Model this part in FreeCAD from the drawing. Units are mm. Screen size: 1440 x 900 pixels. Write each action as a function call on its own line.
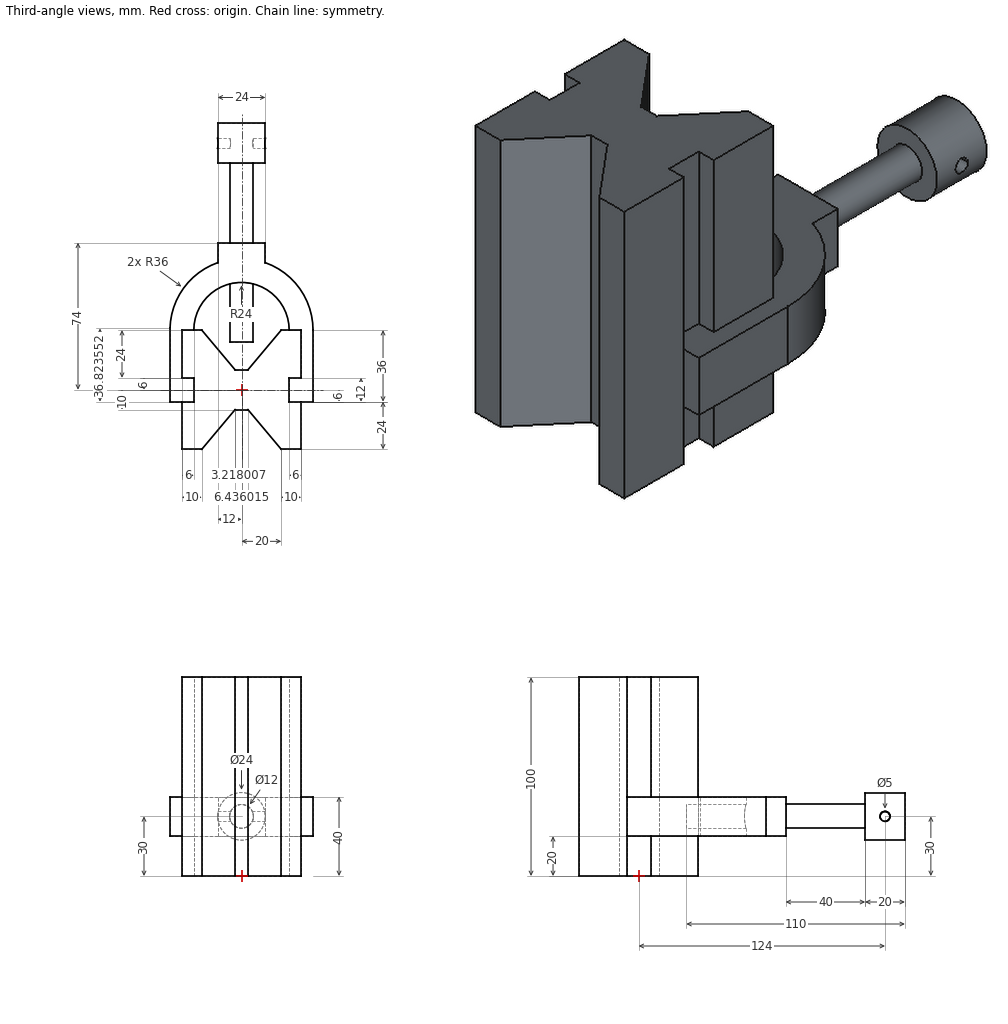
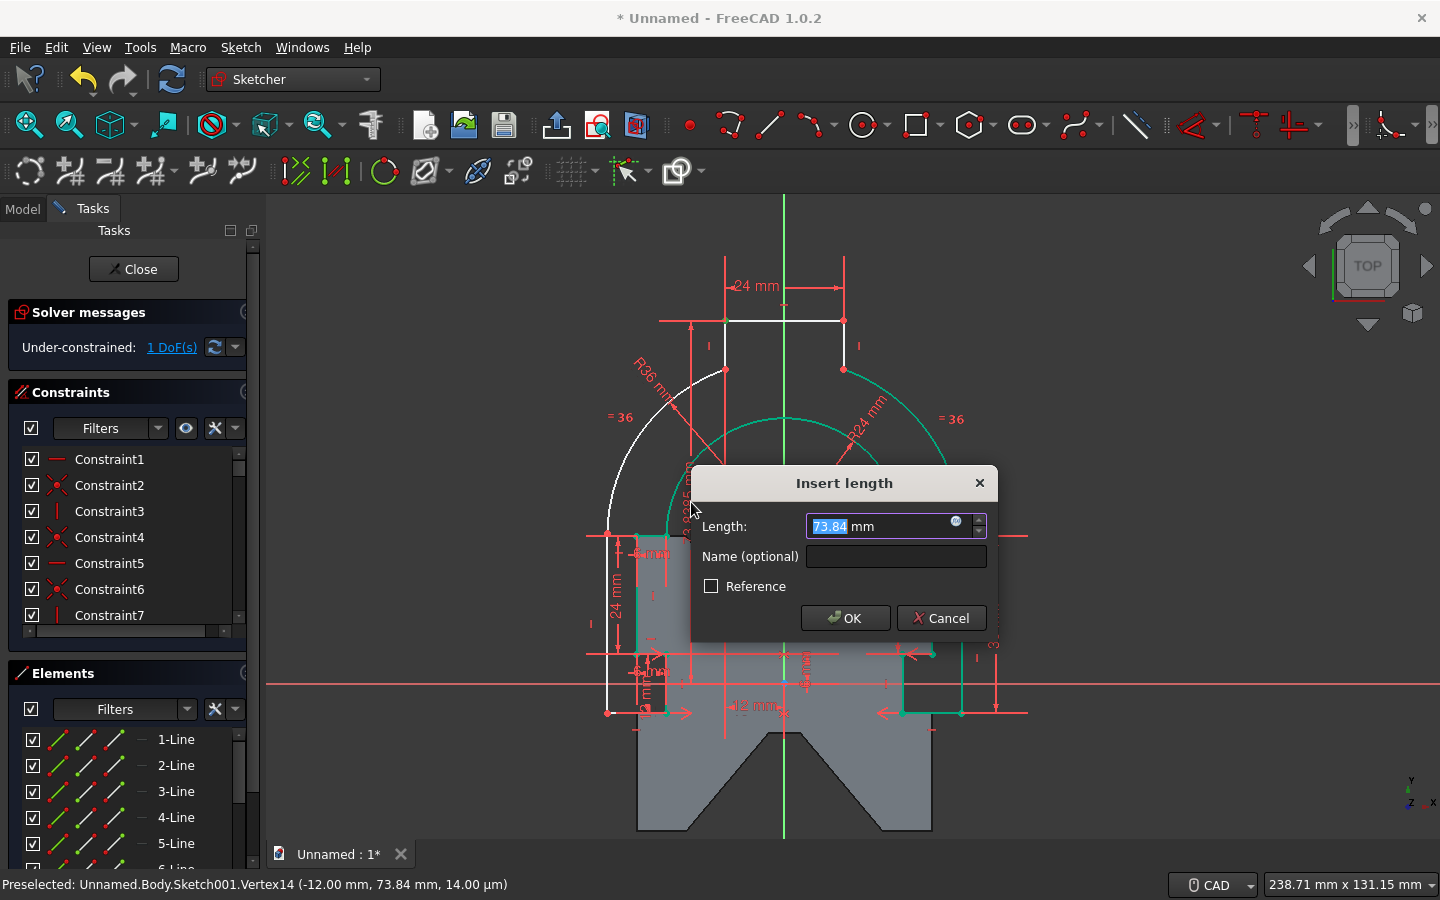
text(74)
key(Return)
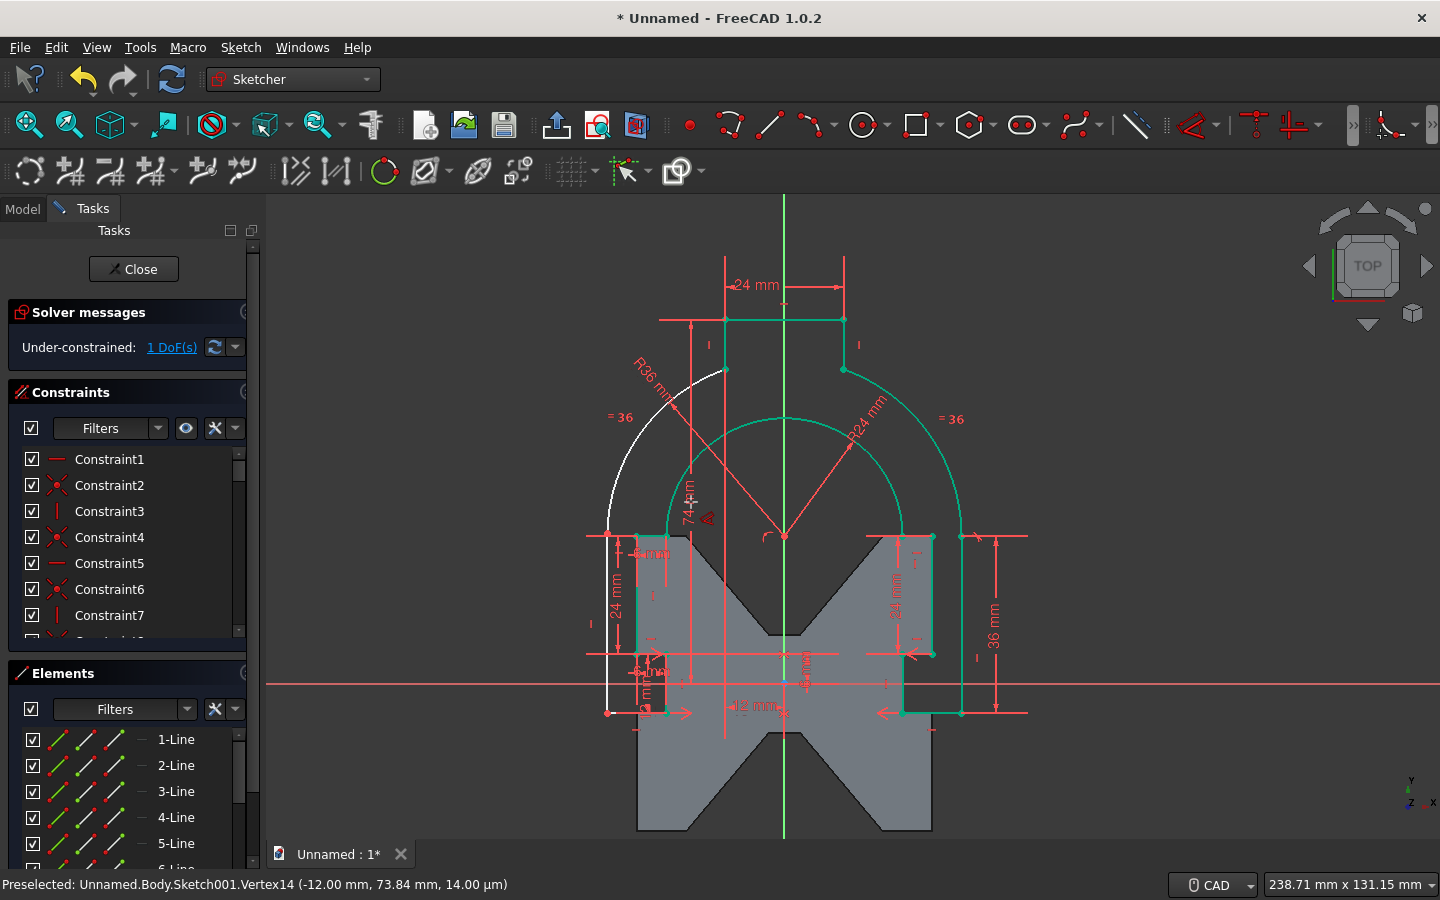
click(607, 659)
click(573, 624)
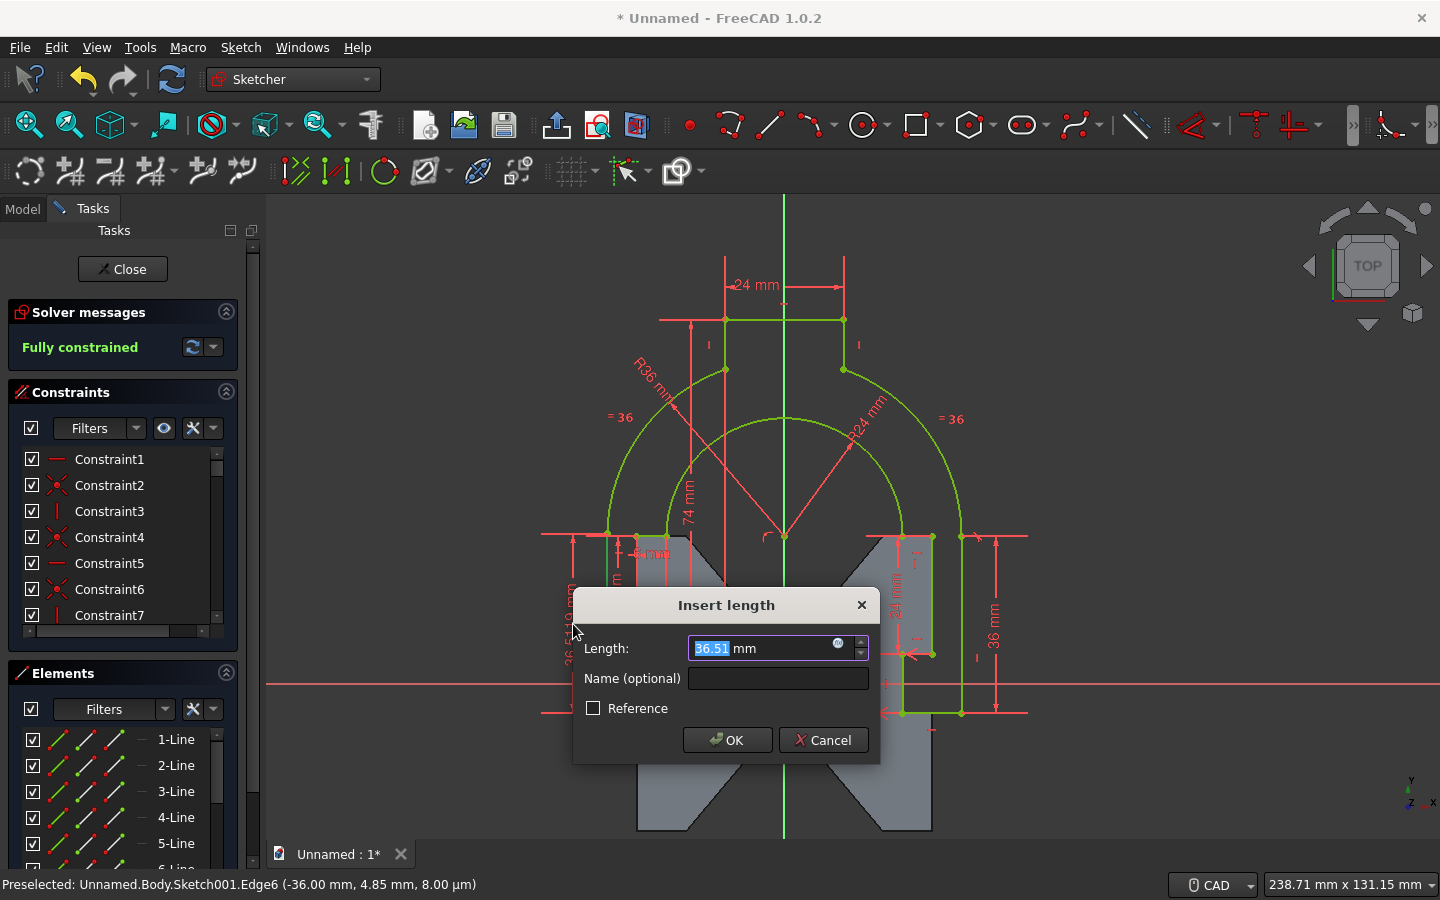
text(36.823552)
key(Return)
key(Escape)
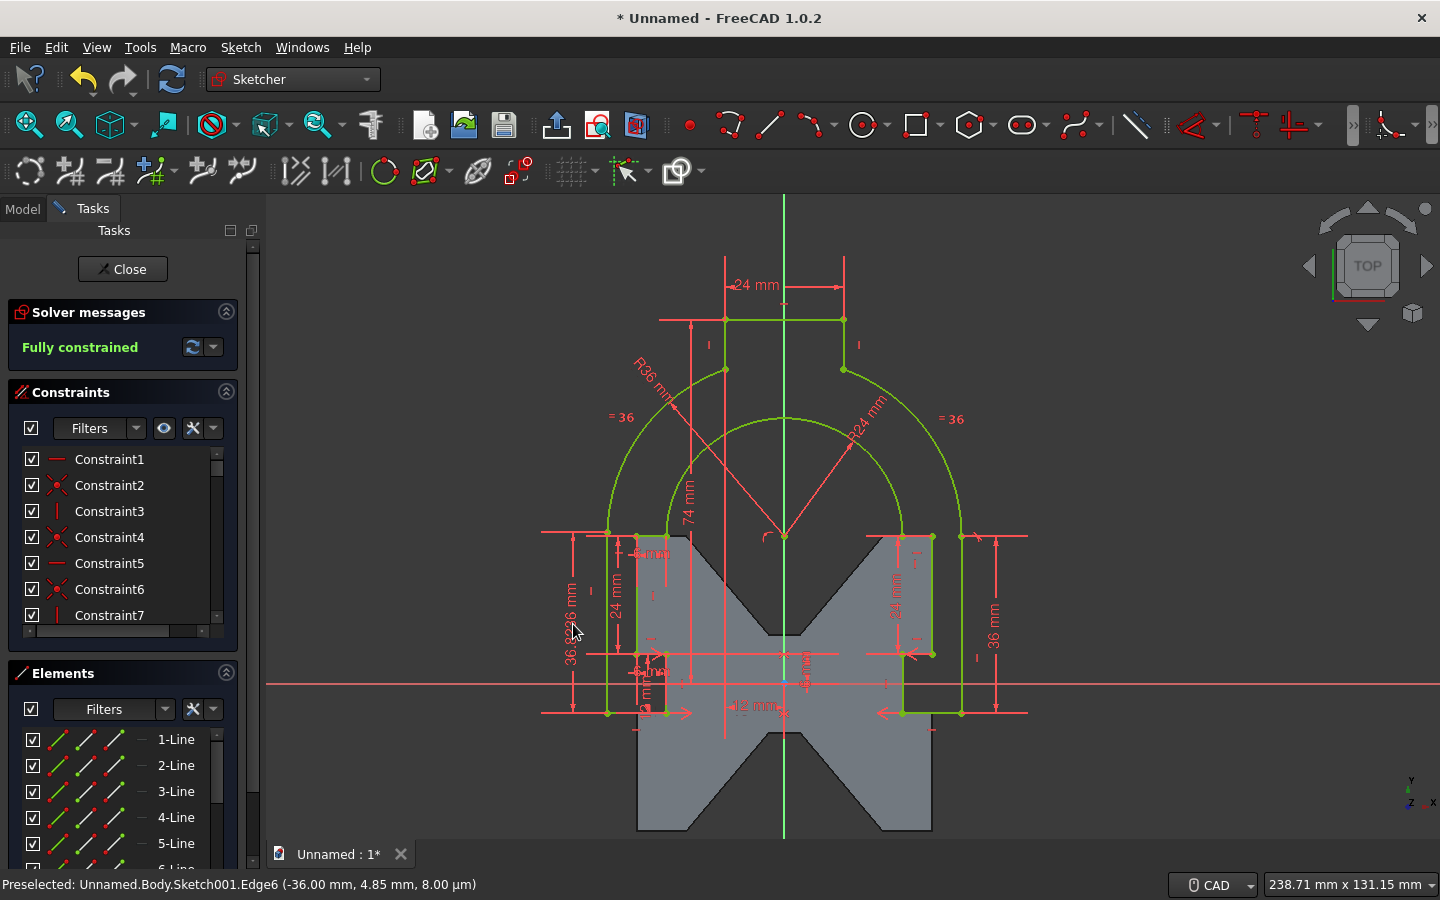
click(123, 269)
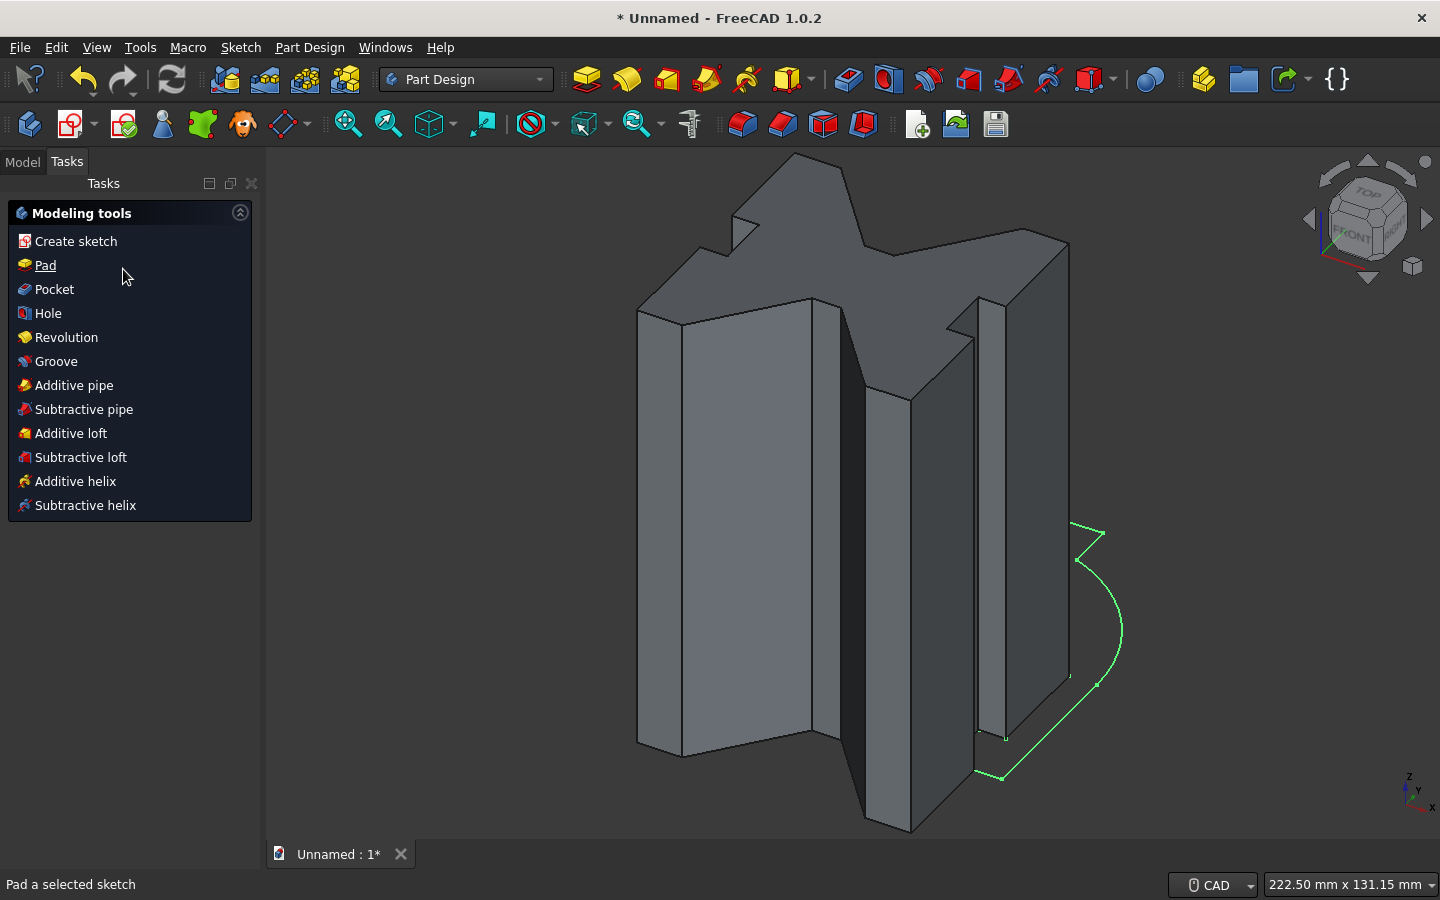
click(588, 80)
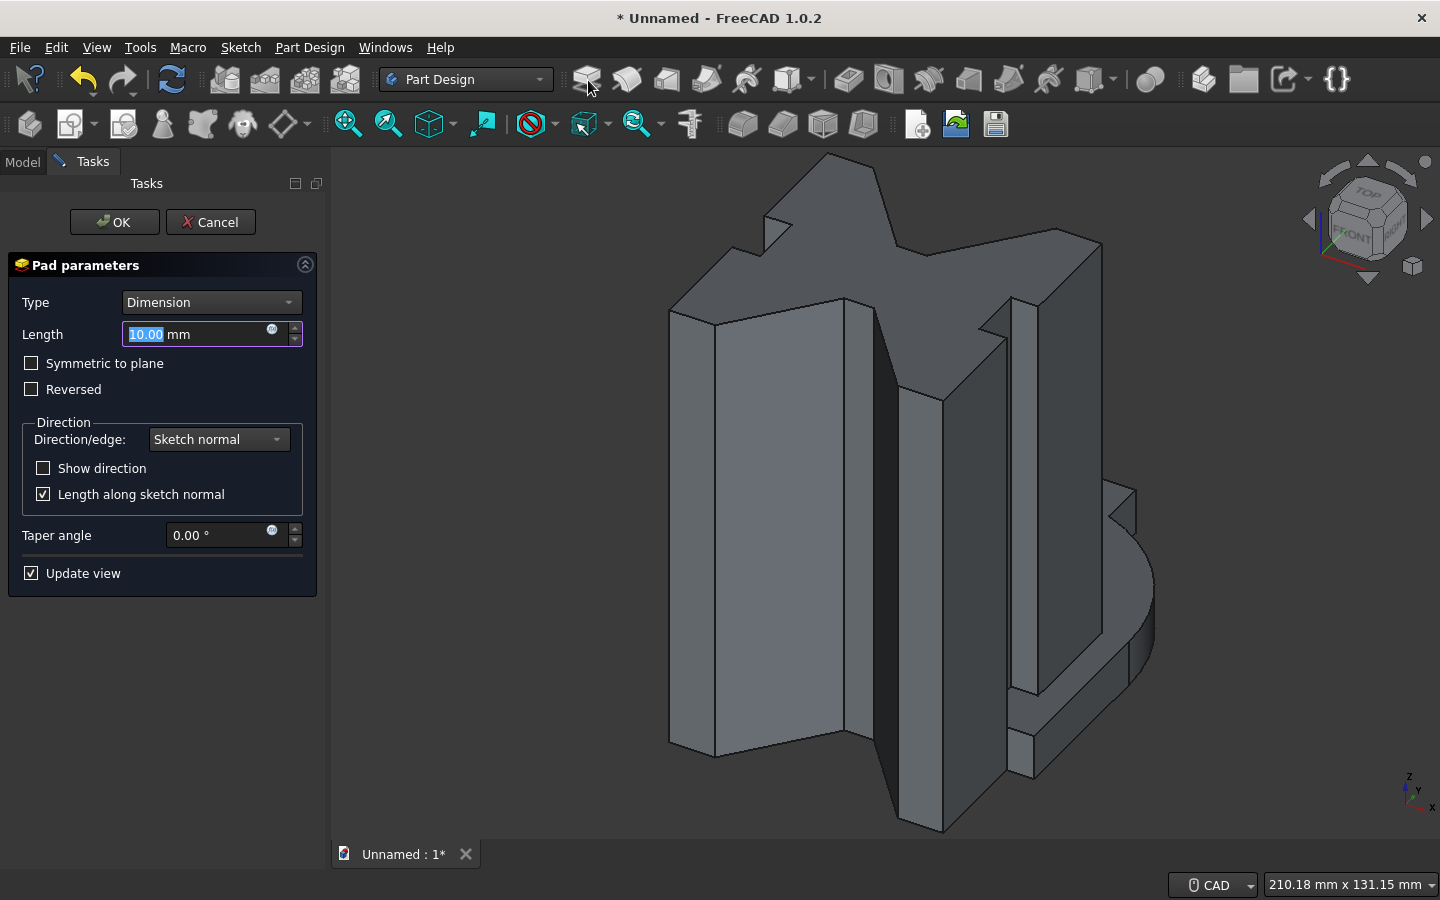
text(40)
key(Tab)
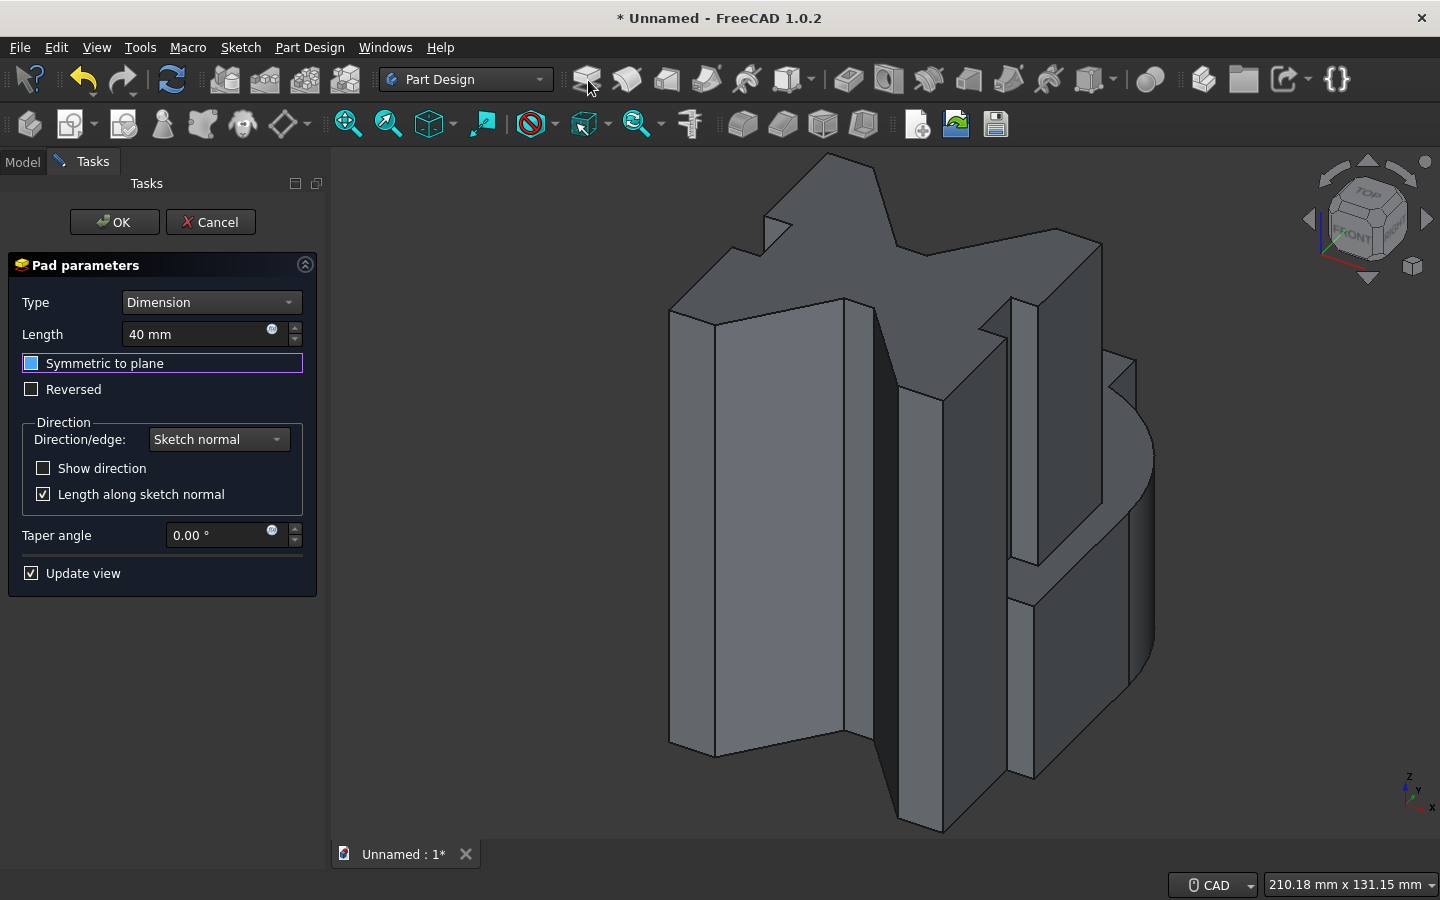
click(115, 222)